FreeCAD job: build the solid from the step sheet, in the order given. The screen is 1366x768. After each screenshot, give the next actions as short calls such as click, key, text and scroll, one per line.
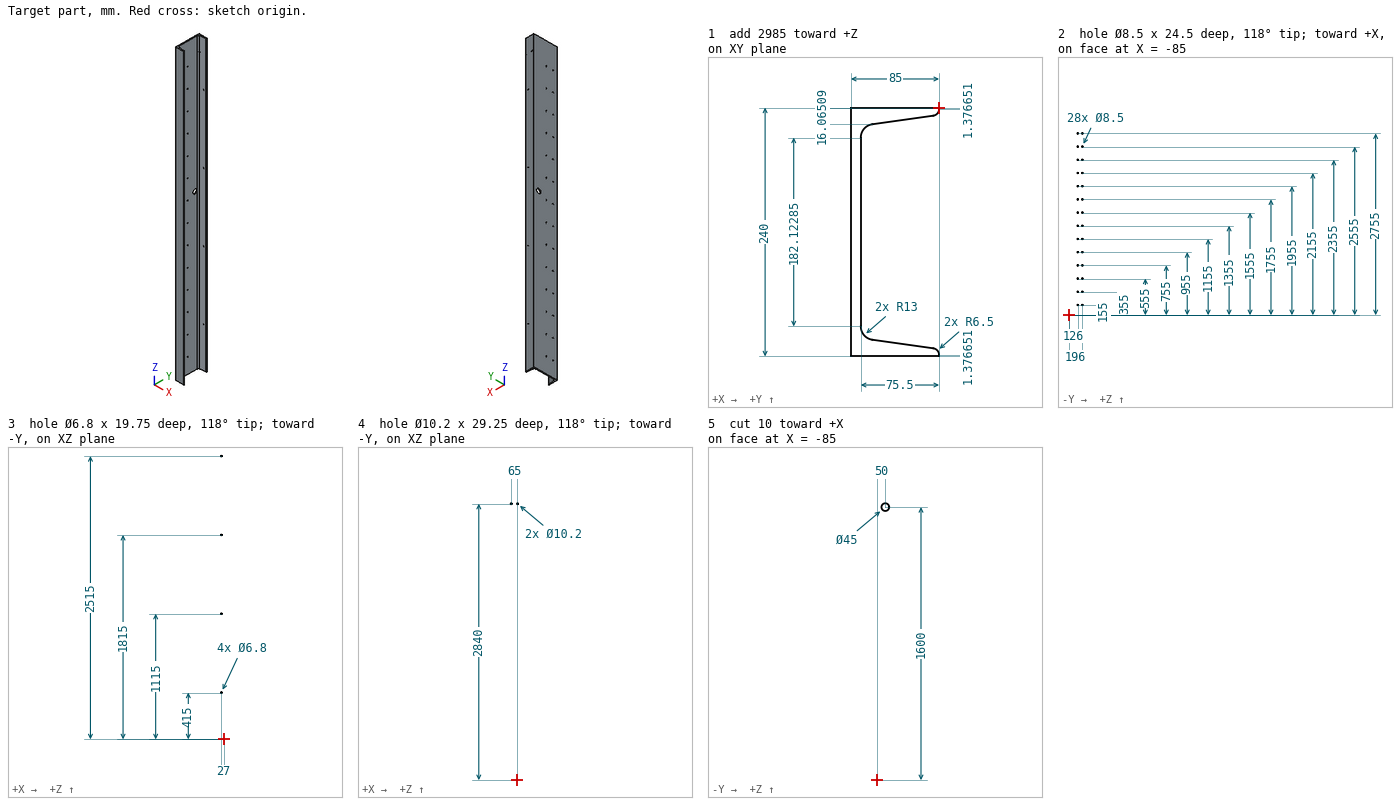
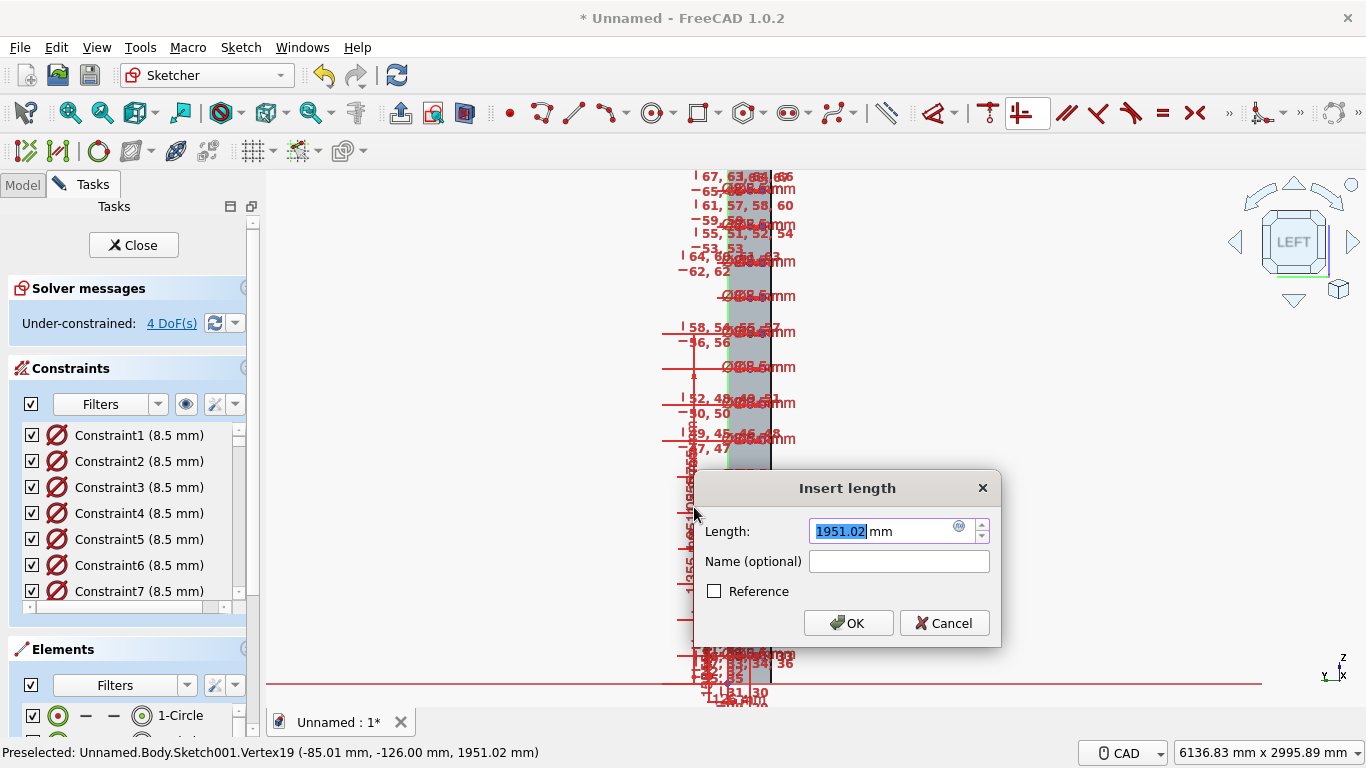
text(1955)
key(Return)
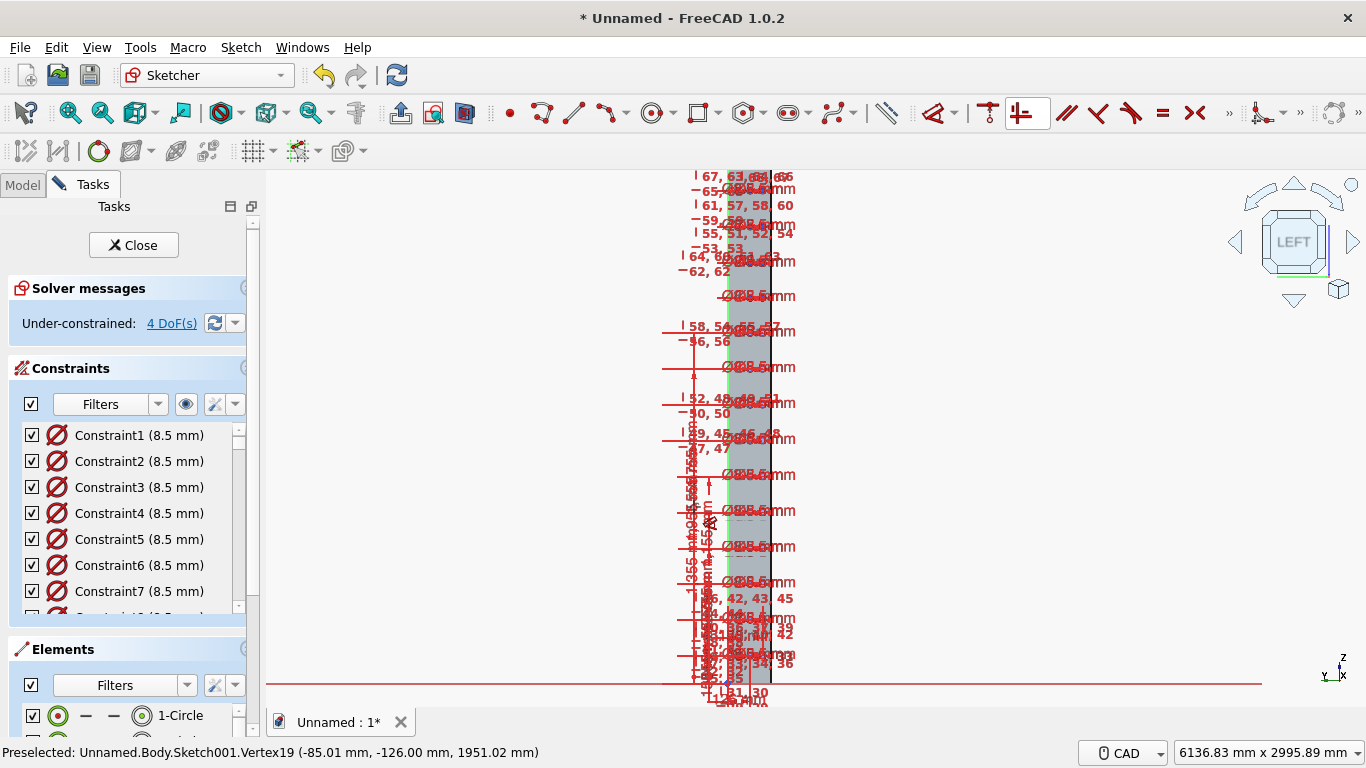
click(763, 298)
click(694, 401)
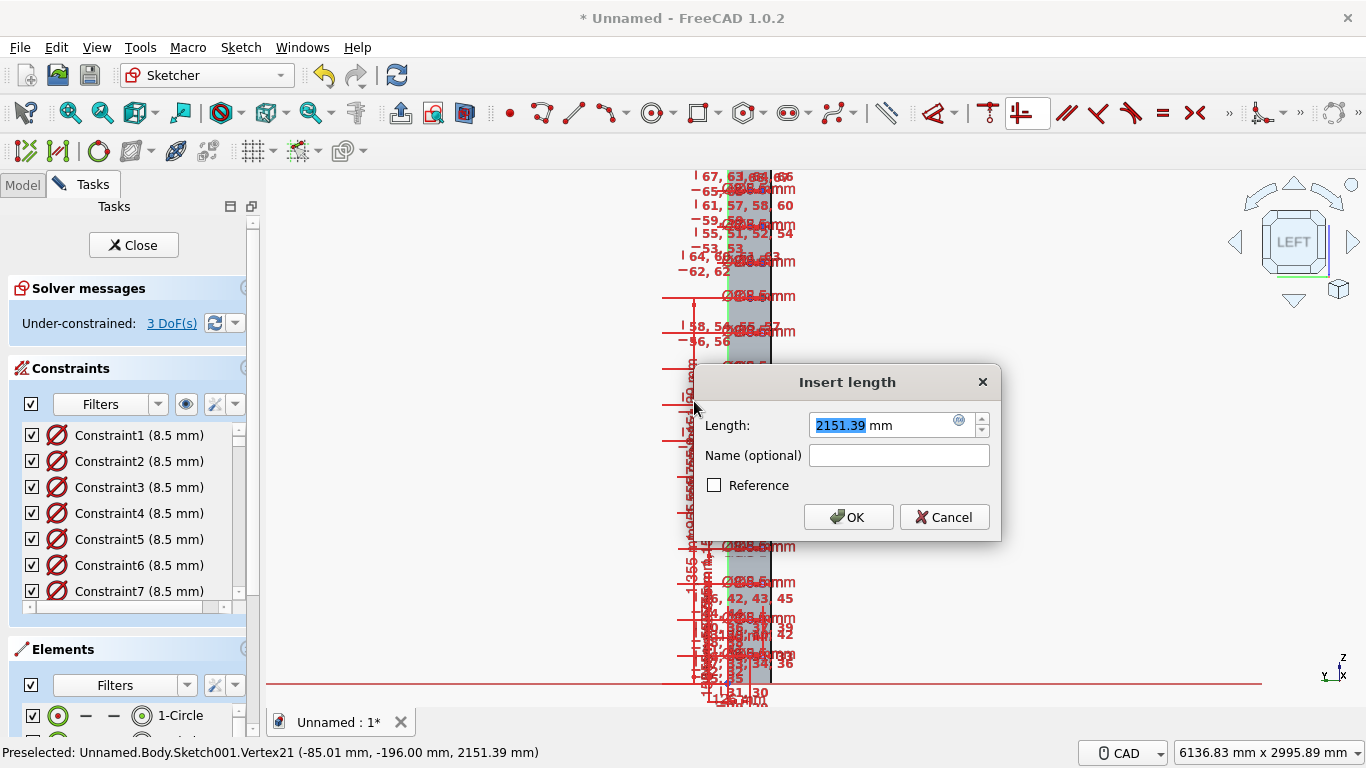
text(2155)
key(Return)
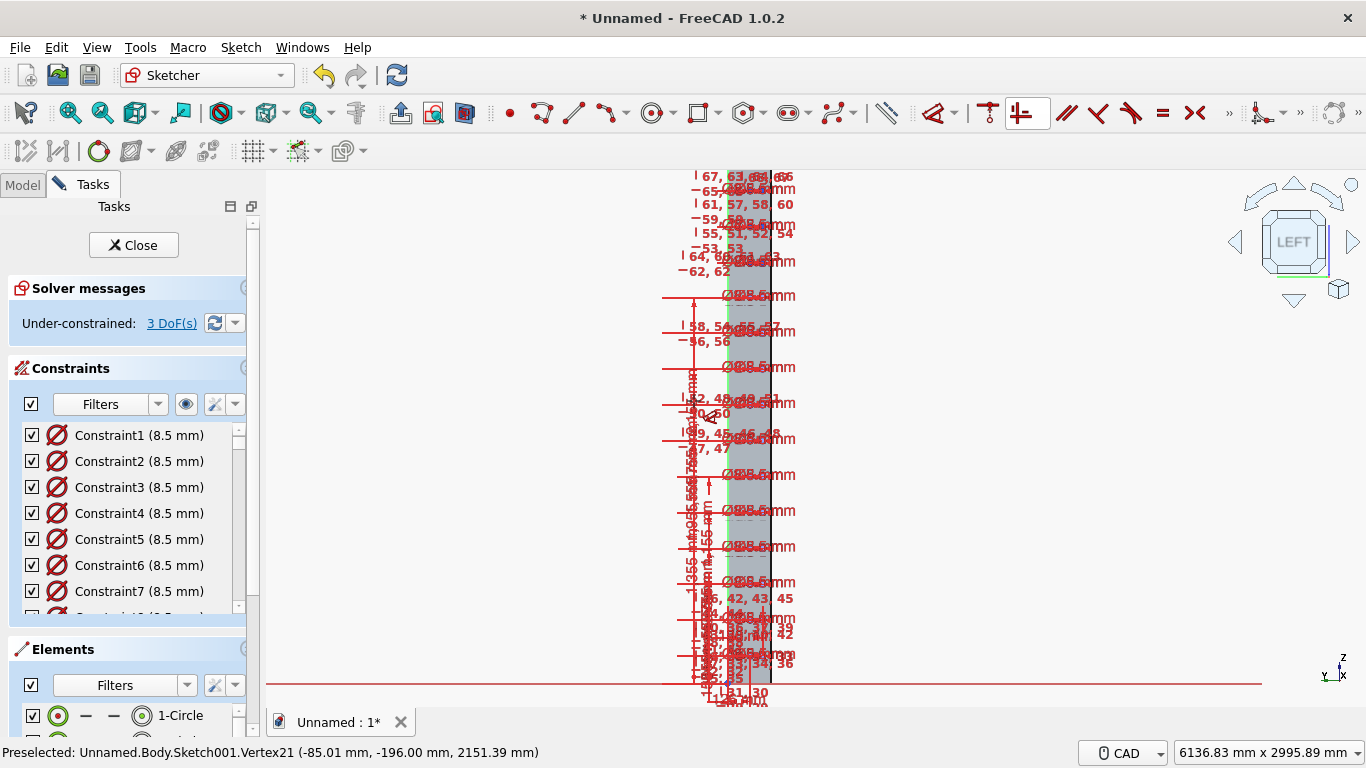
click(750, 263)
click(694, 376)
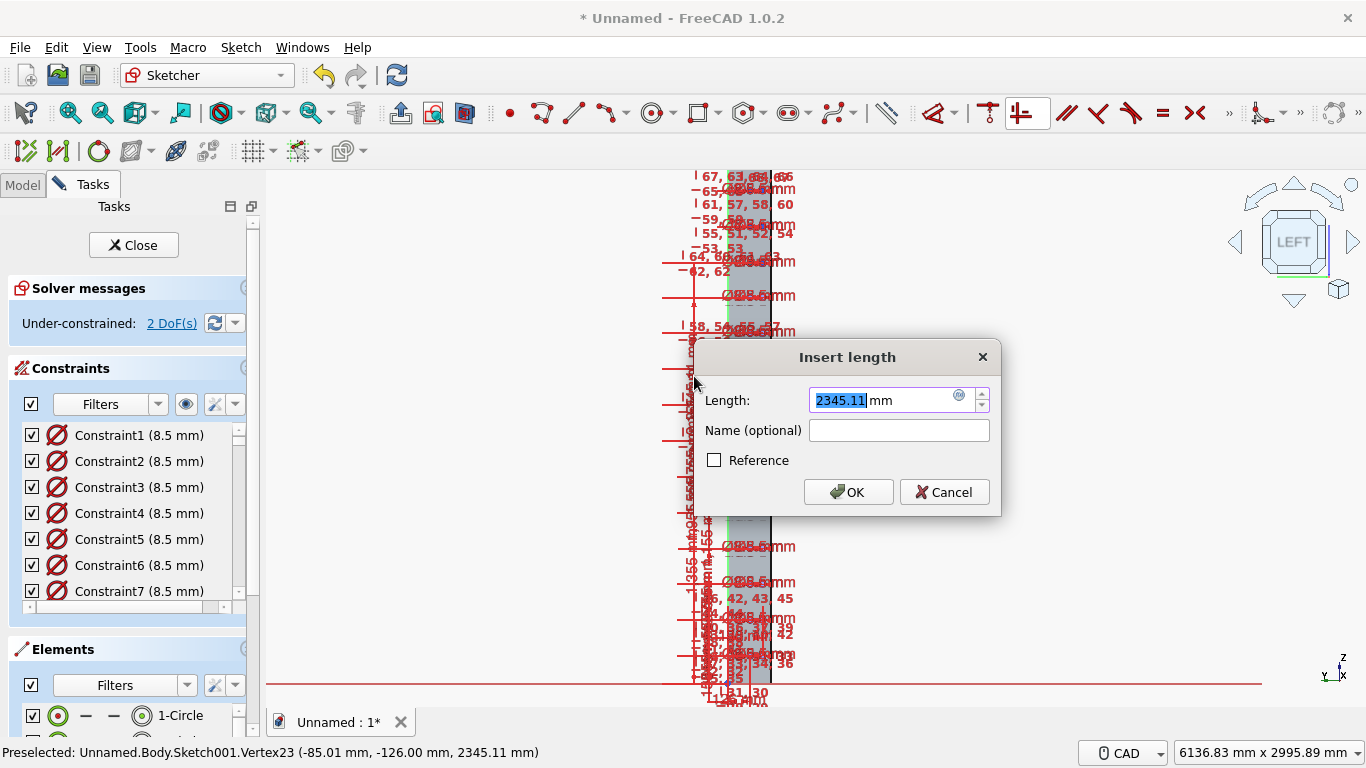
text(2355)
key(Return)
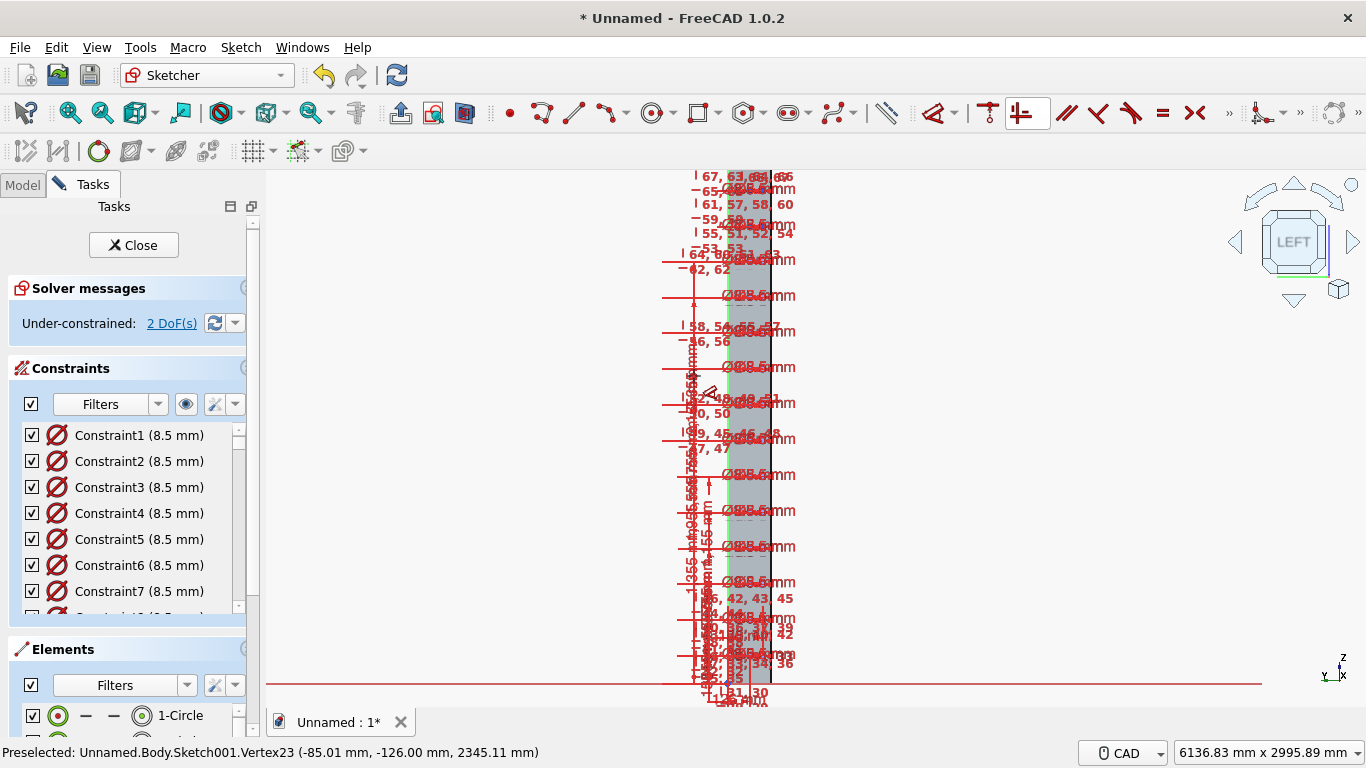
click(763, 227)
click(694, 349)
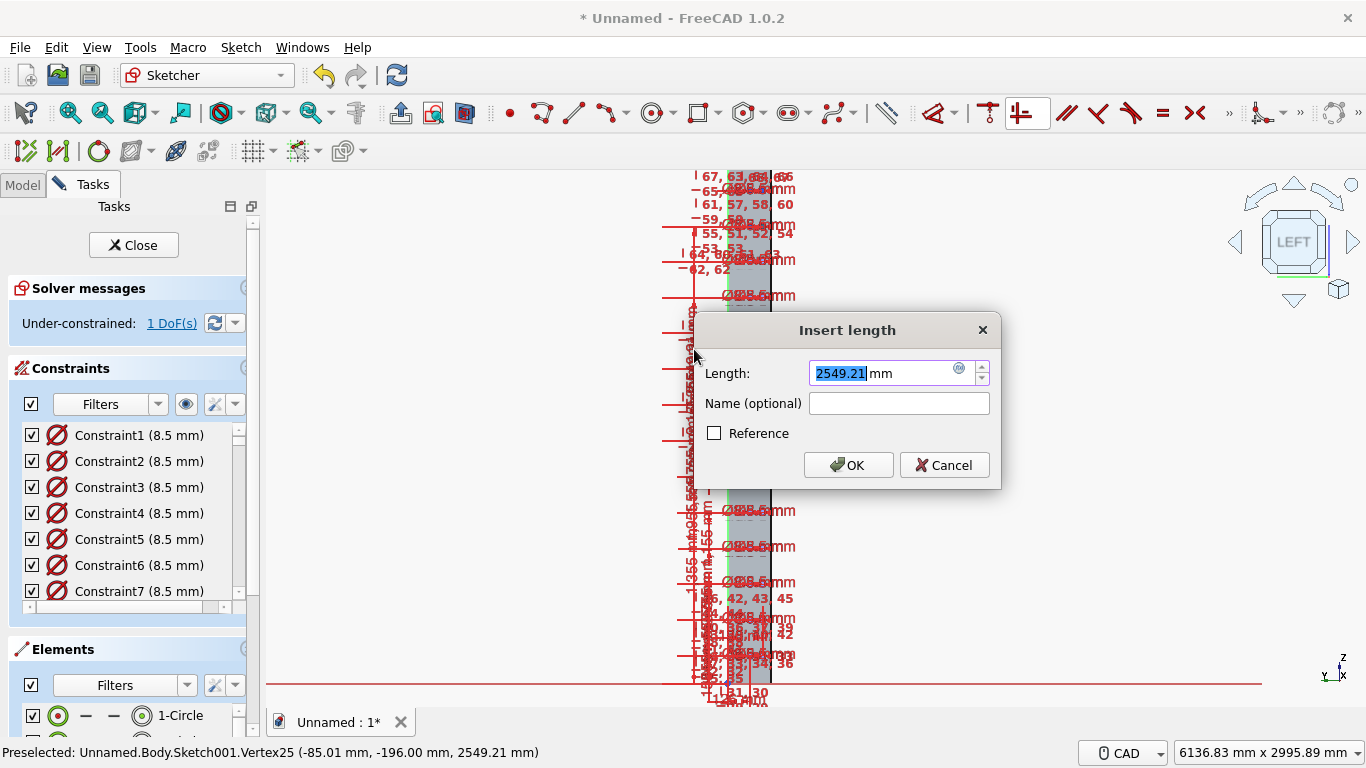
text(2555)
key(Return)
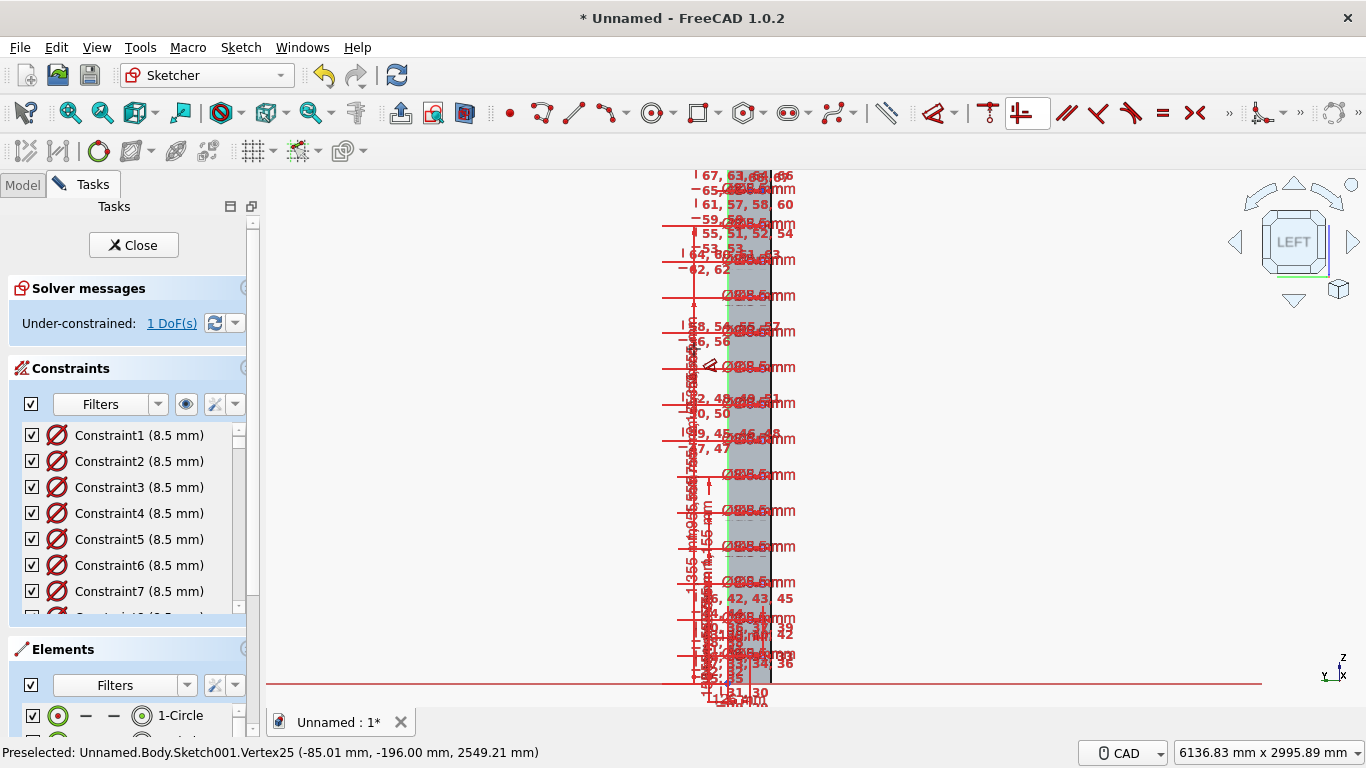
scroll(751, 442, down, 2)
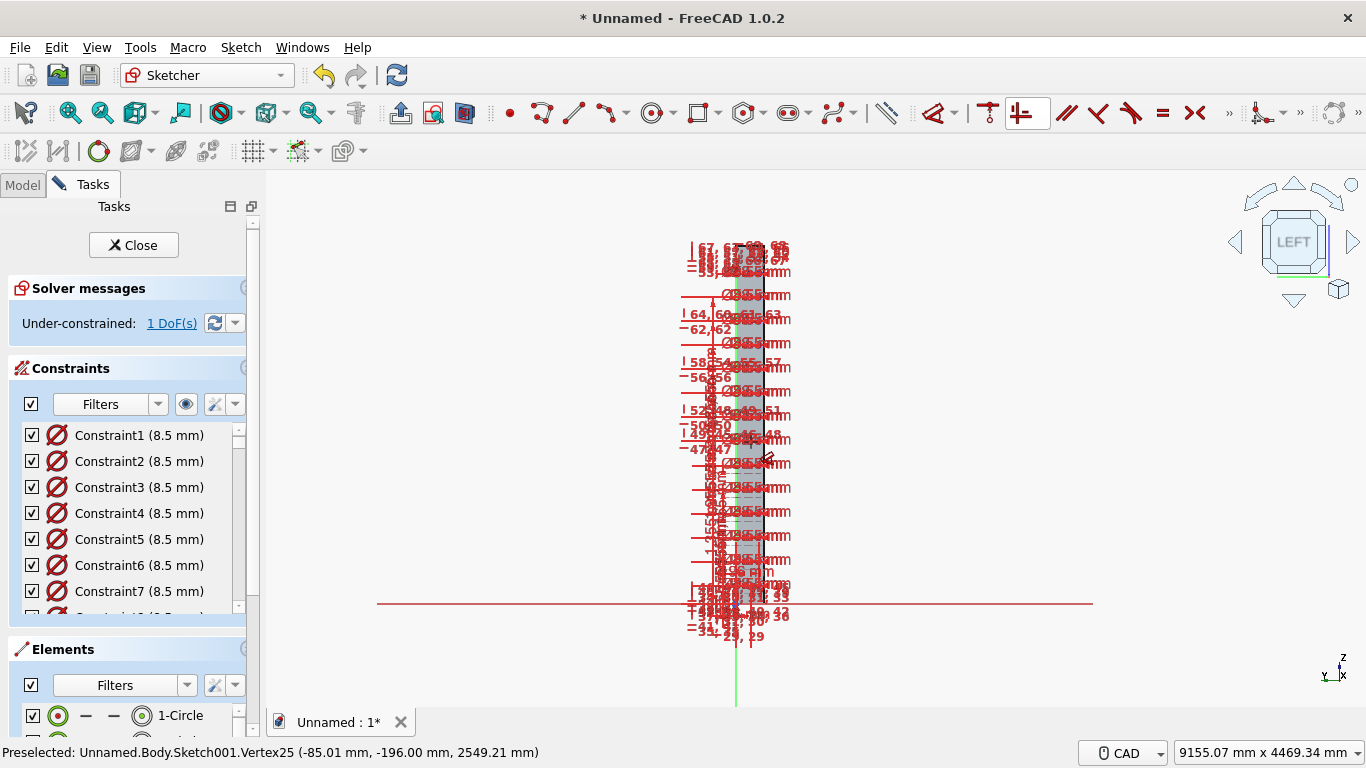
scroll(751, 274, up, 2)